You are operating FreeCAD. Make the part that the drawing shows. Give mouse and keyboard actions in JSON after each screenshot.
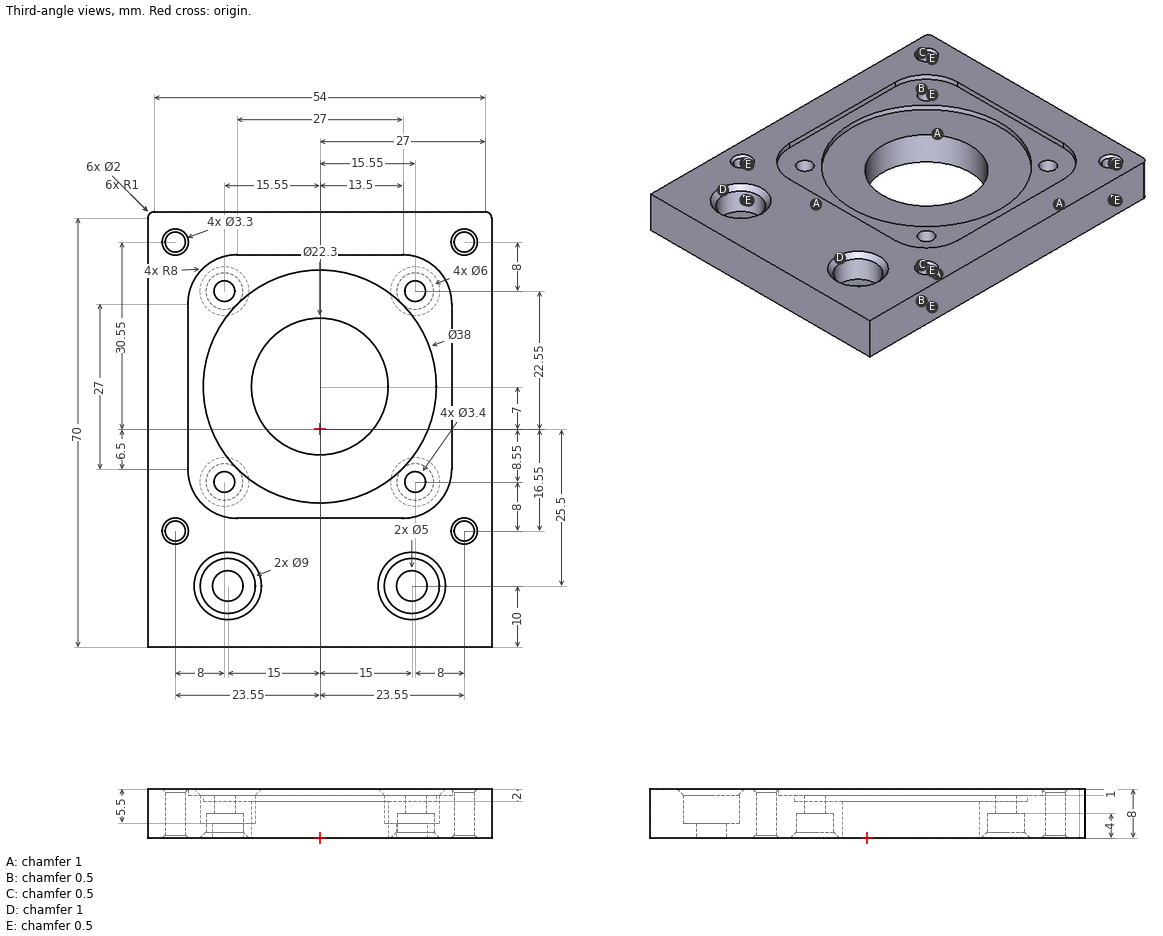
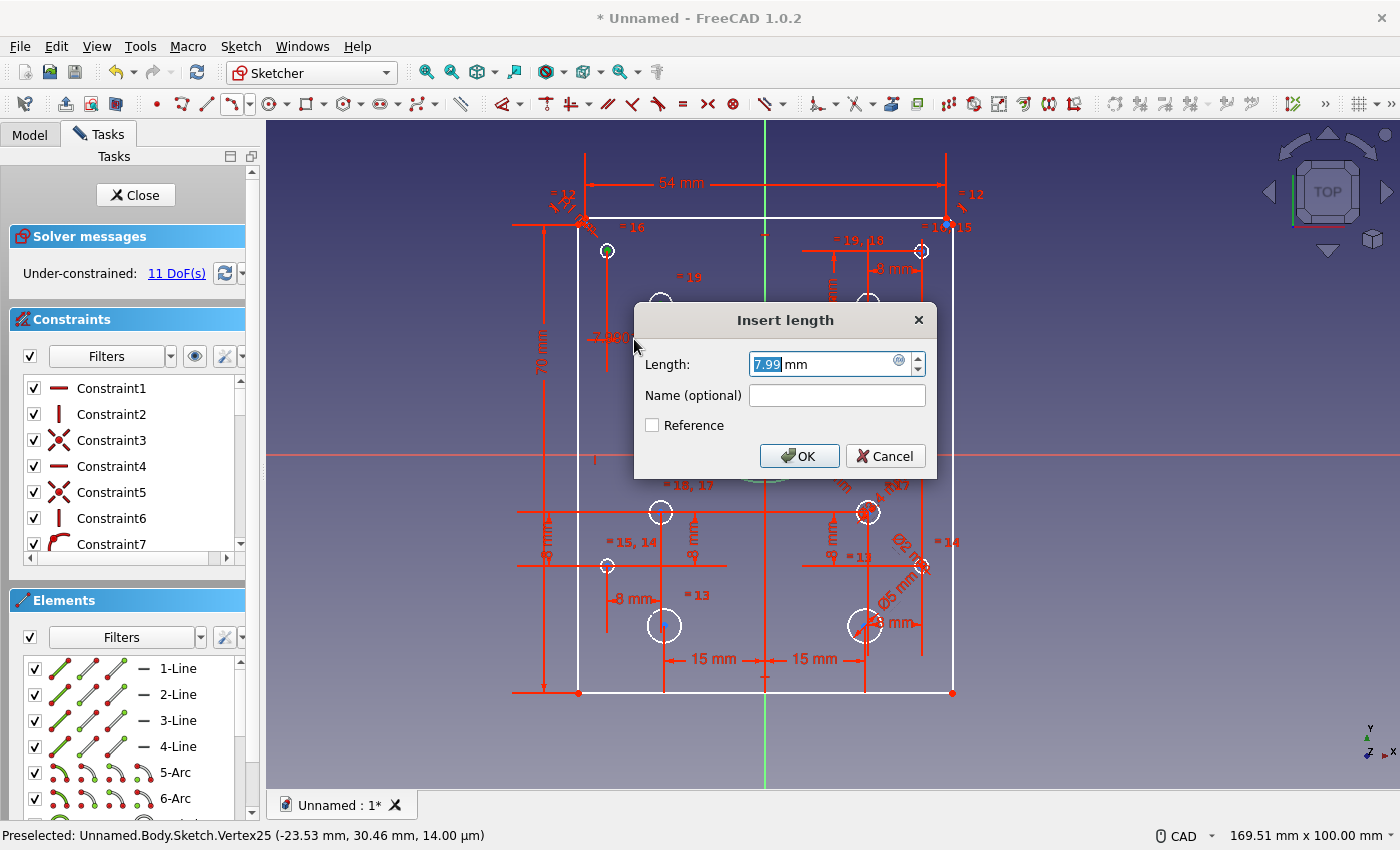
{"action": "type", "text": "8"}
{"action": "key", "text": "Return"}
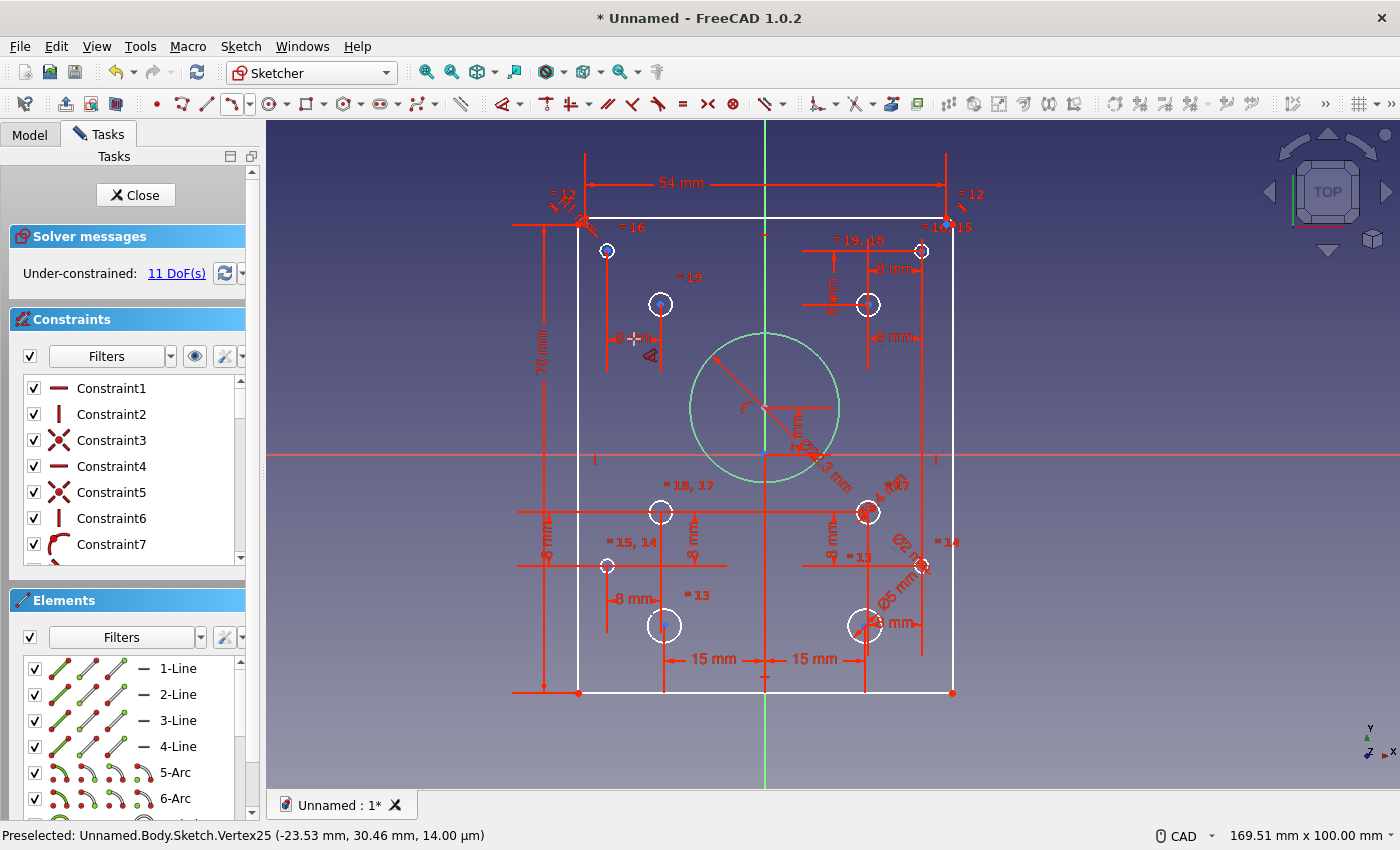
{"action": "left_click", "coordinate": [661, 305]}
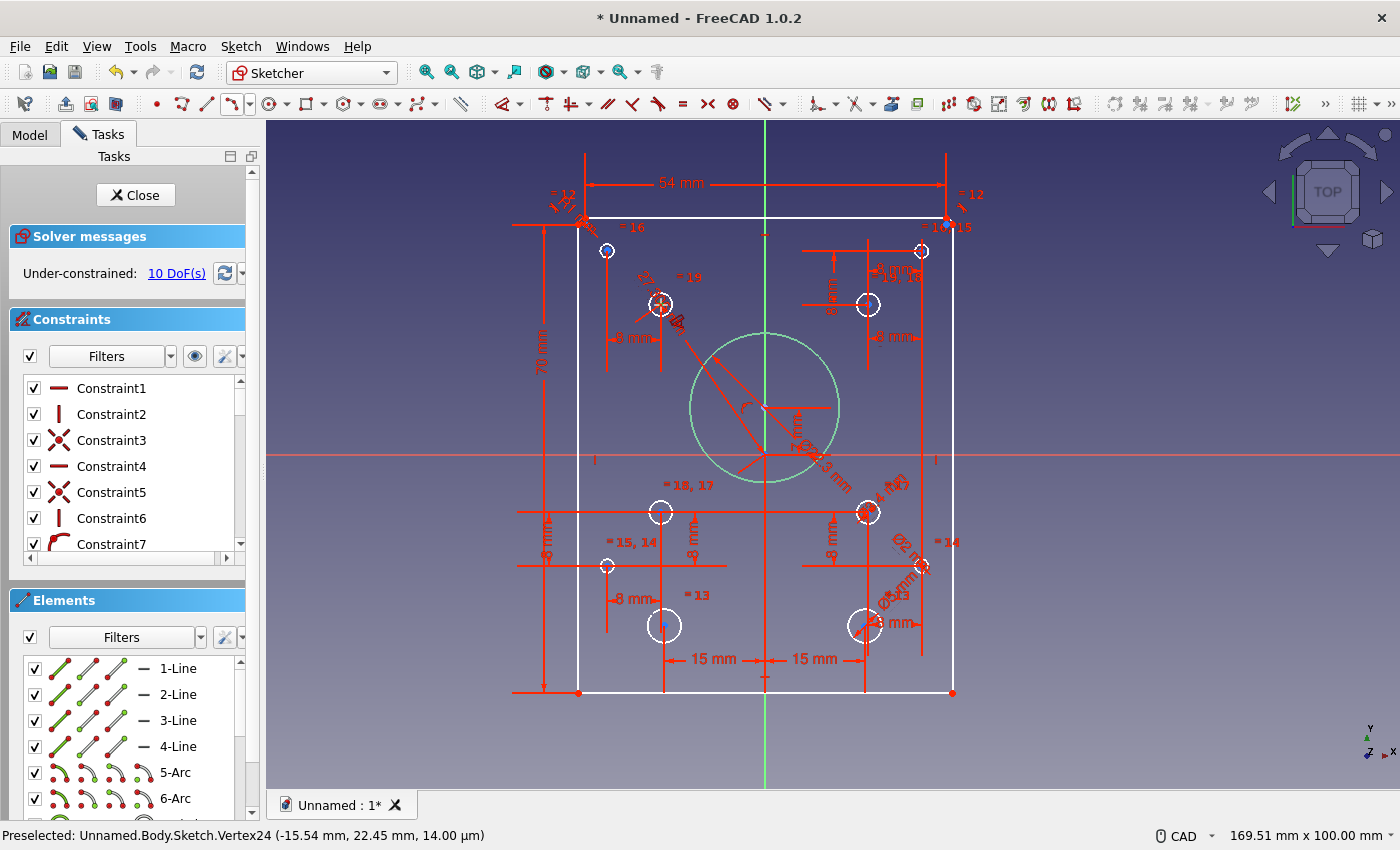
{"action": "left_click", "coordinate": [607, 251]}
{"action": "left_click", "coordinate": [695, 278]}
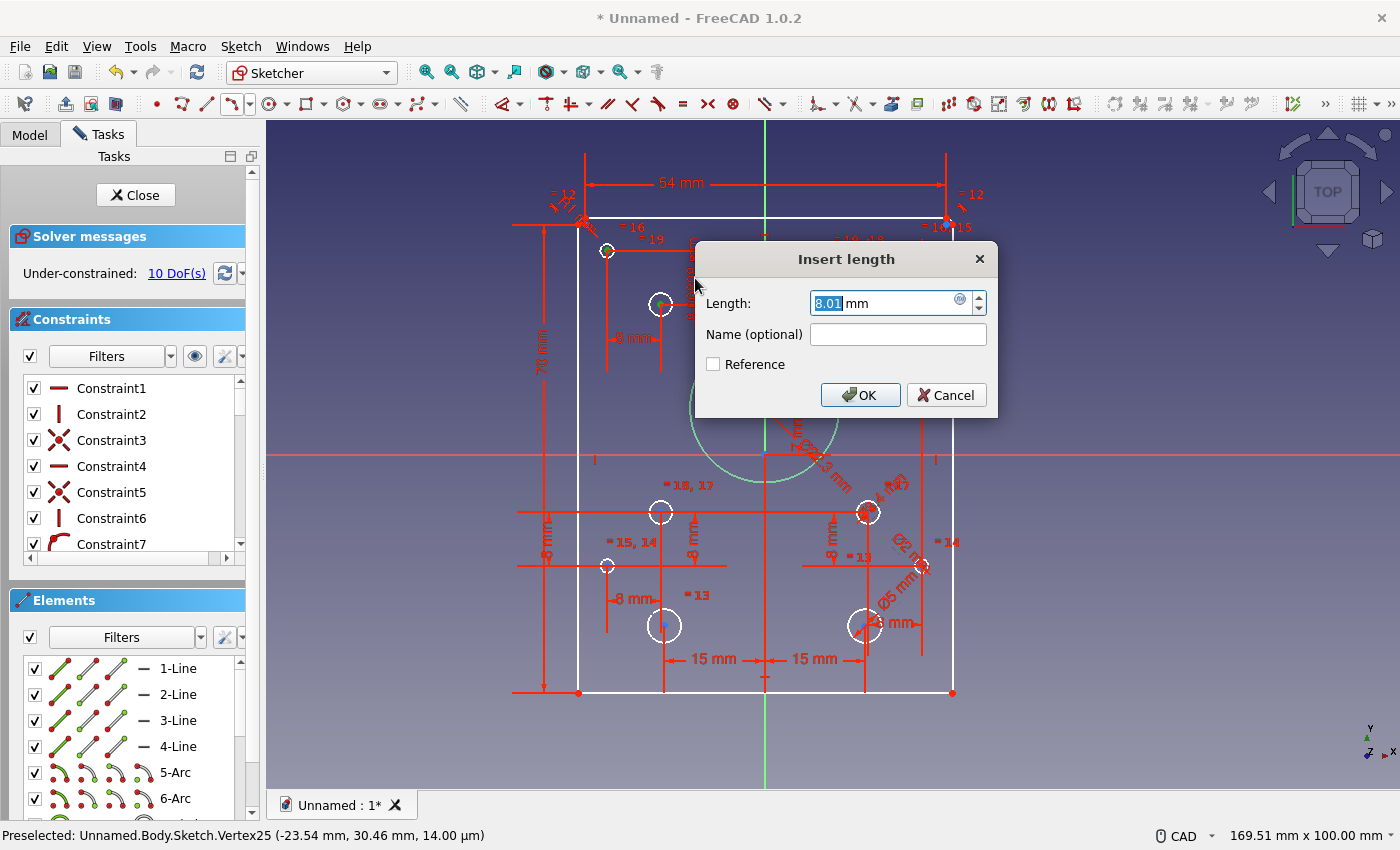
{"action": "type", "text": "8"}
{"action": "key", "text": "Return"}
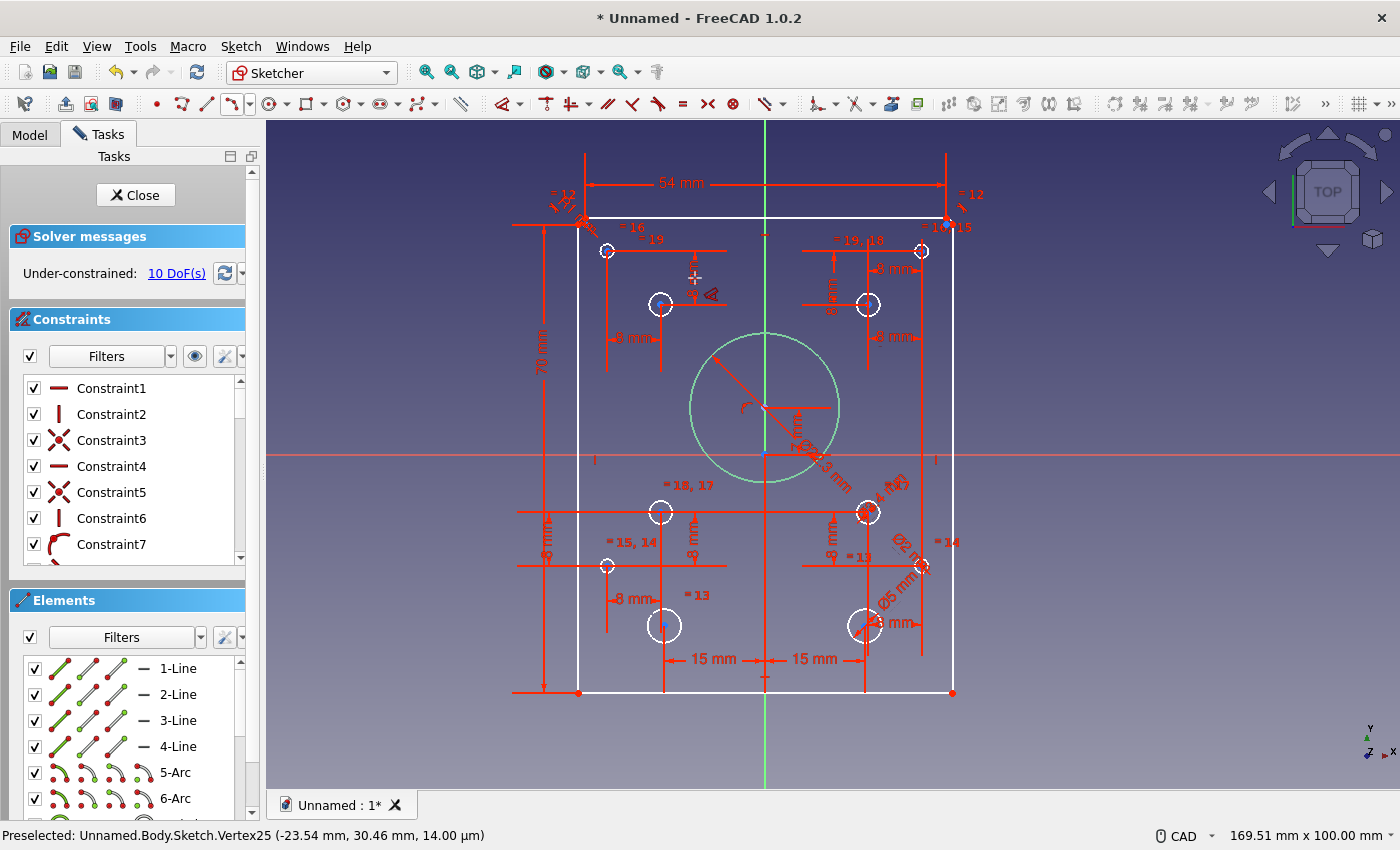
{"action": "scroll", "coordinate": [946, 218], "scroll_direction": "up", "scroll_amount": 4}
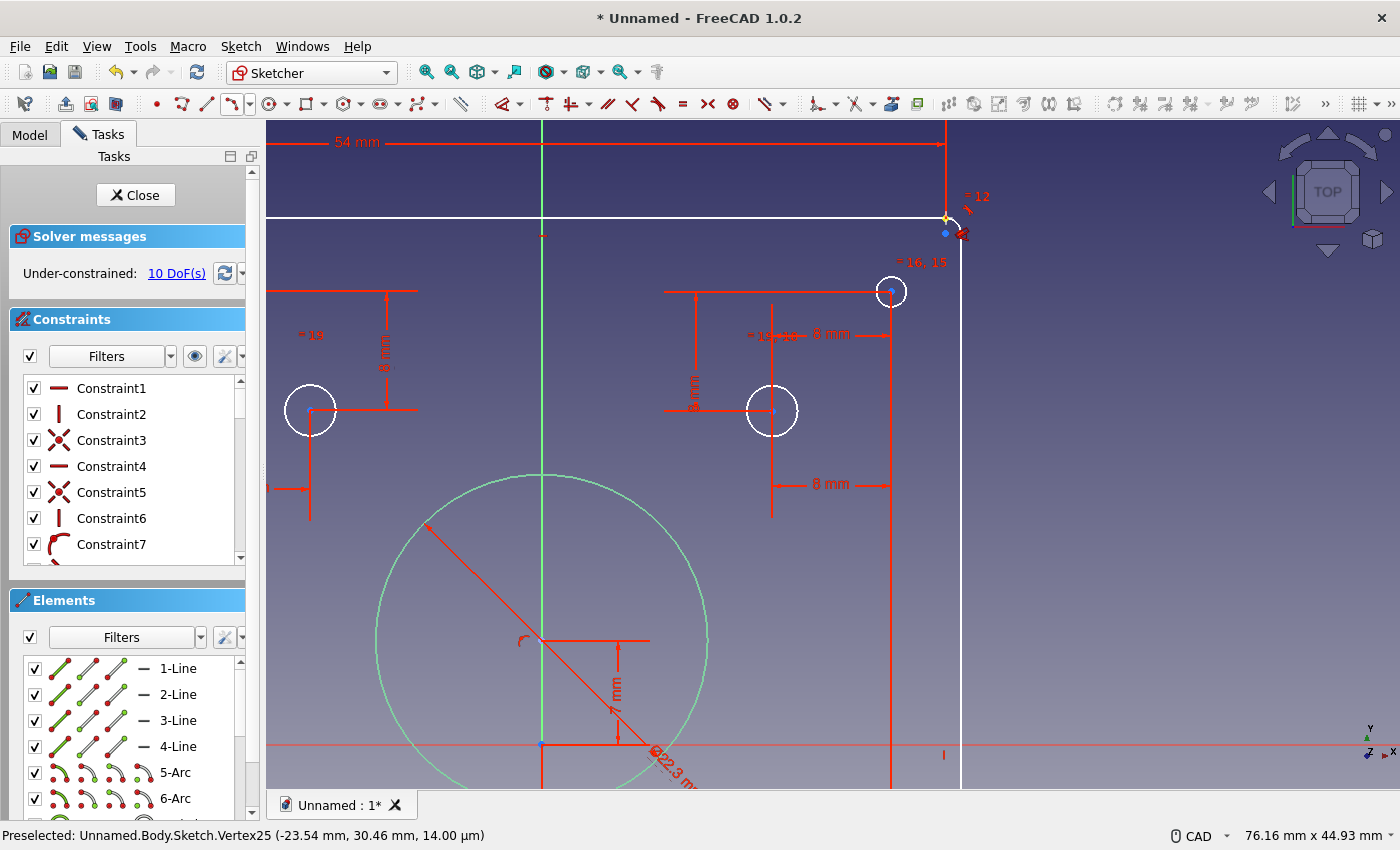
{"action": "left_click", "coordinate": [946, 218]}
{"action": "left_click", "coordinate": [744, 184]}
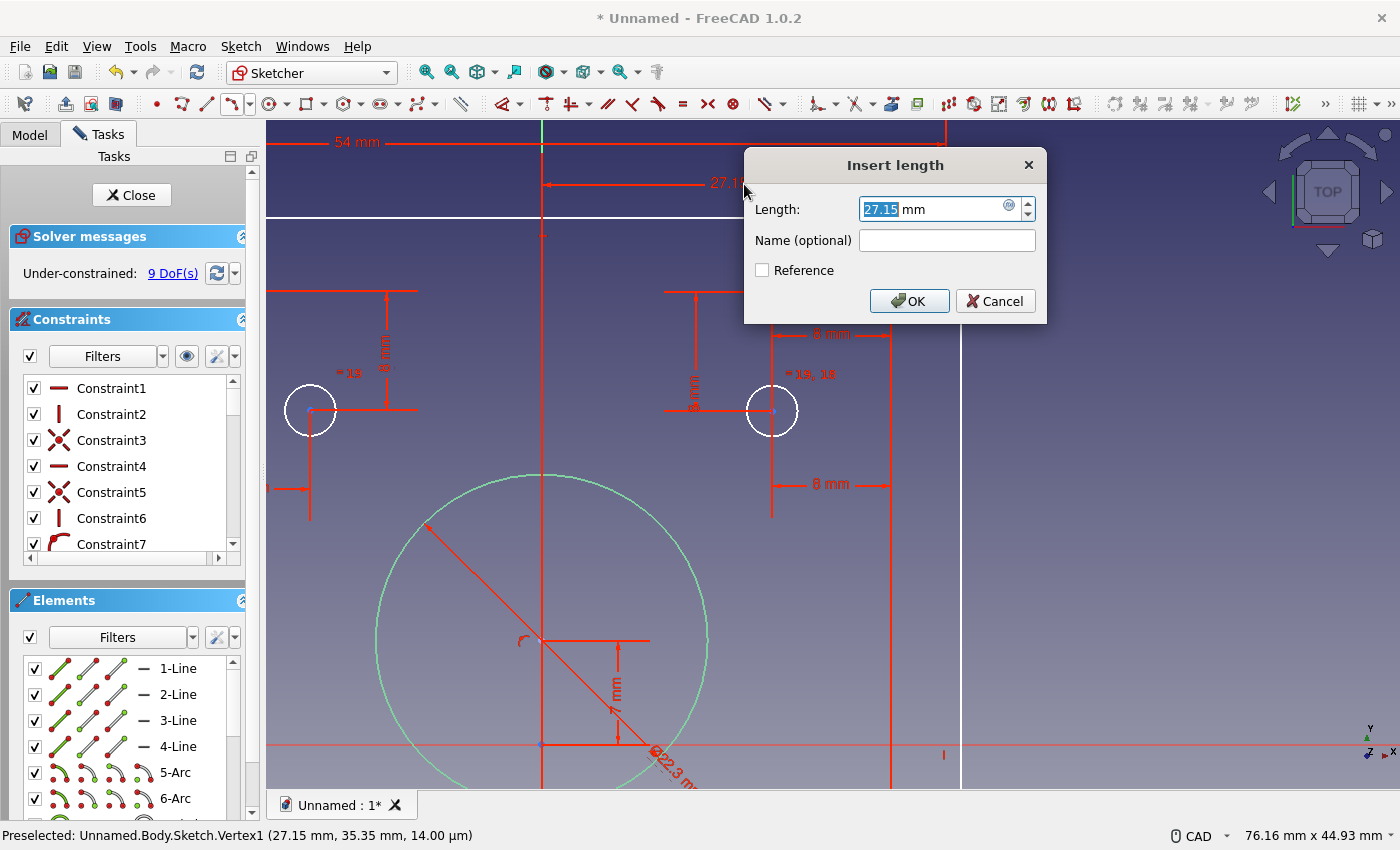
{"action": "type", "text": "27"}
{"action": "key", "text": "Return"}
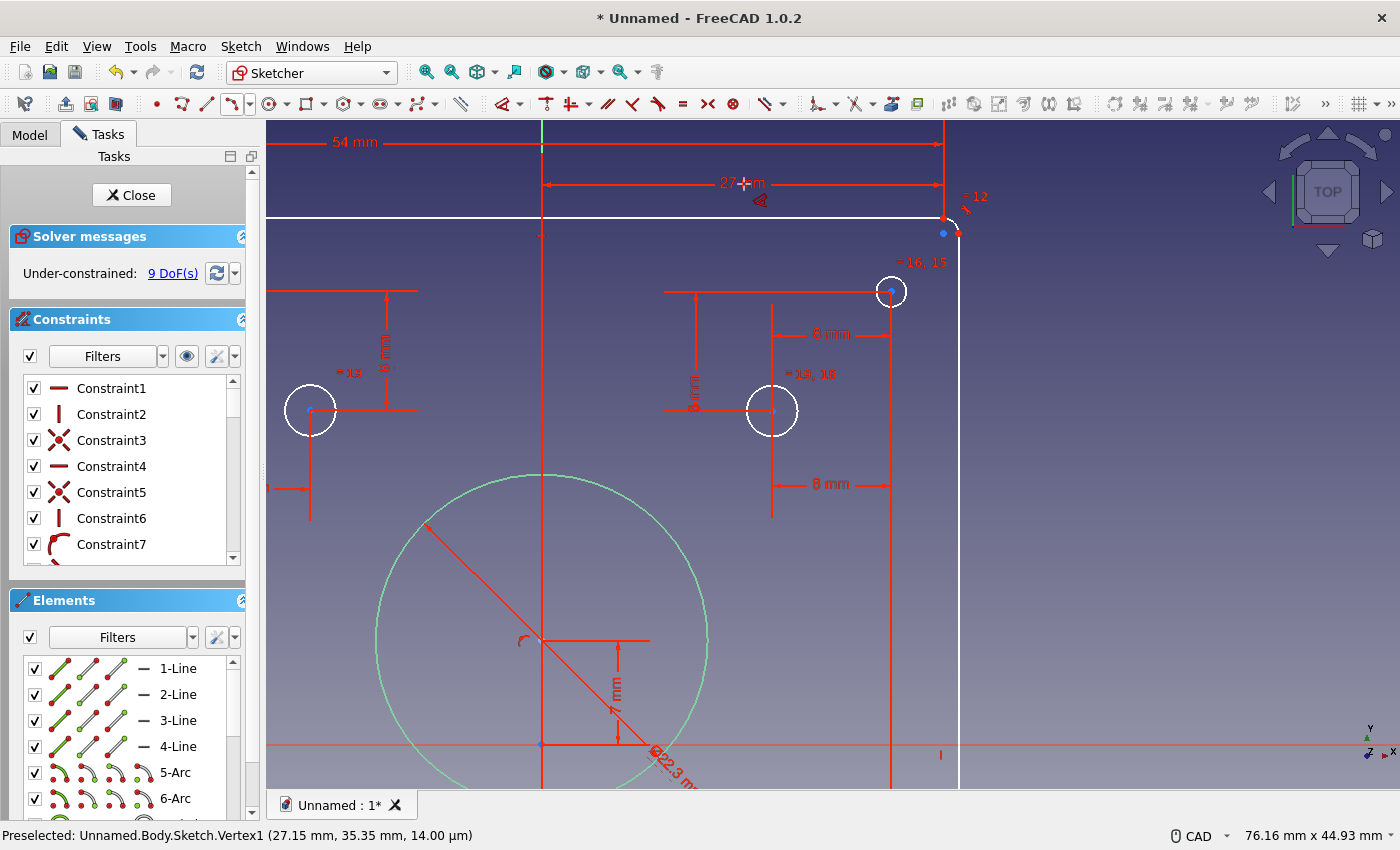
{"action": "scroll", "coordinate": [946, 218], "scroll_direction": "down", "scroll_amount": 4}